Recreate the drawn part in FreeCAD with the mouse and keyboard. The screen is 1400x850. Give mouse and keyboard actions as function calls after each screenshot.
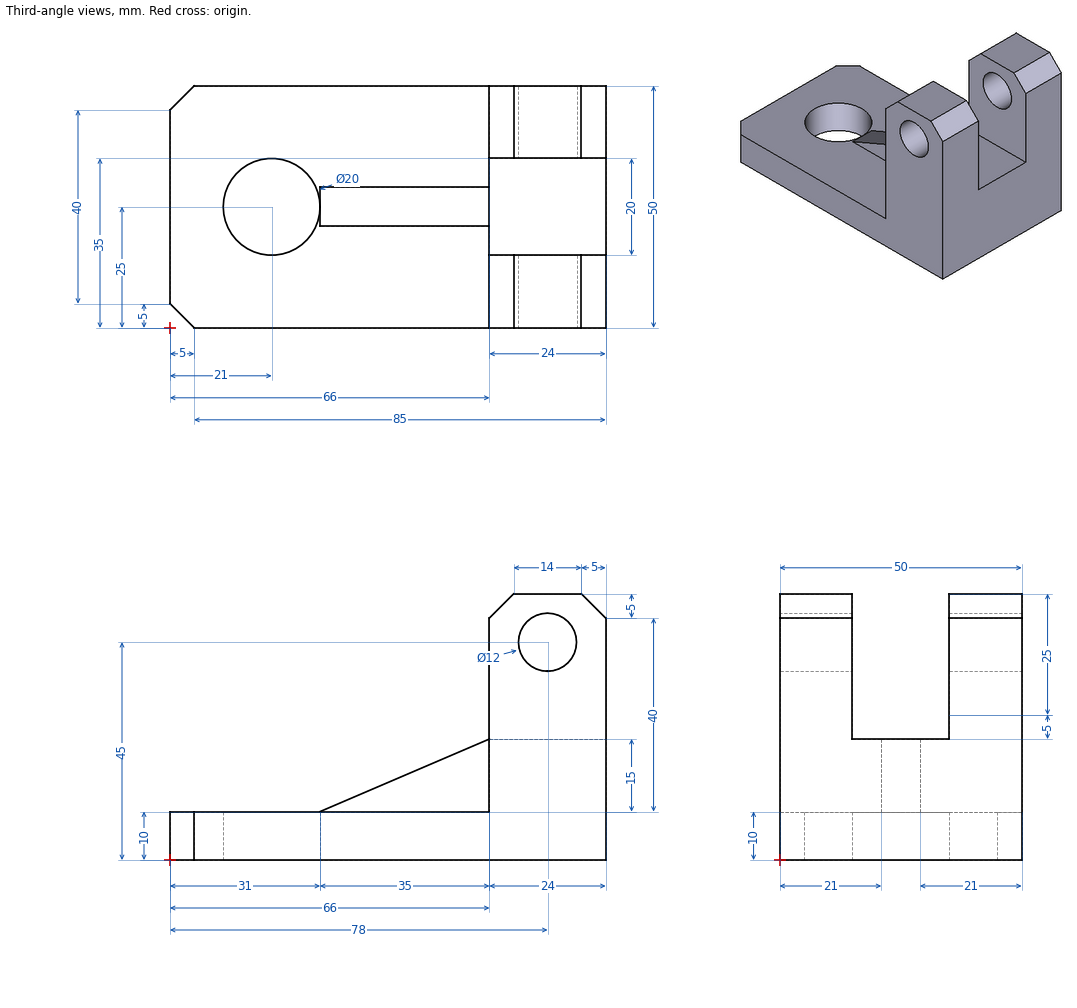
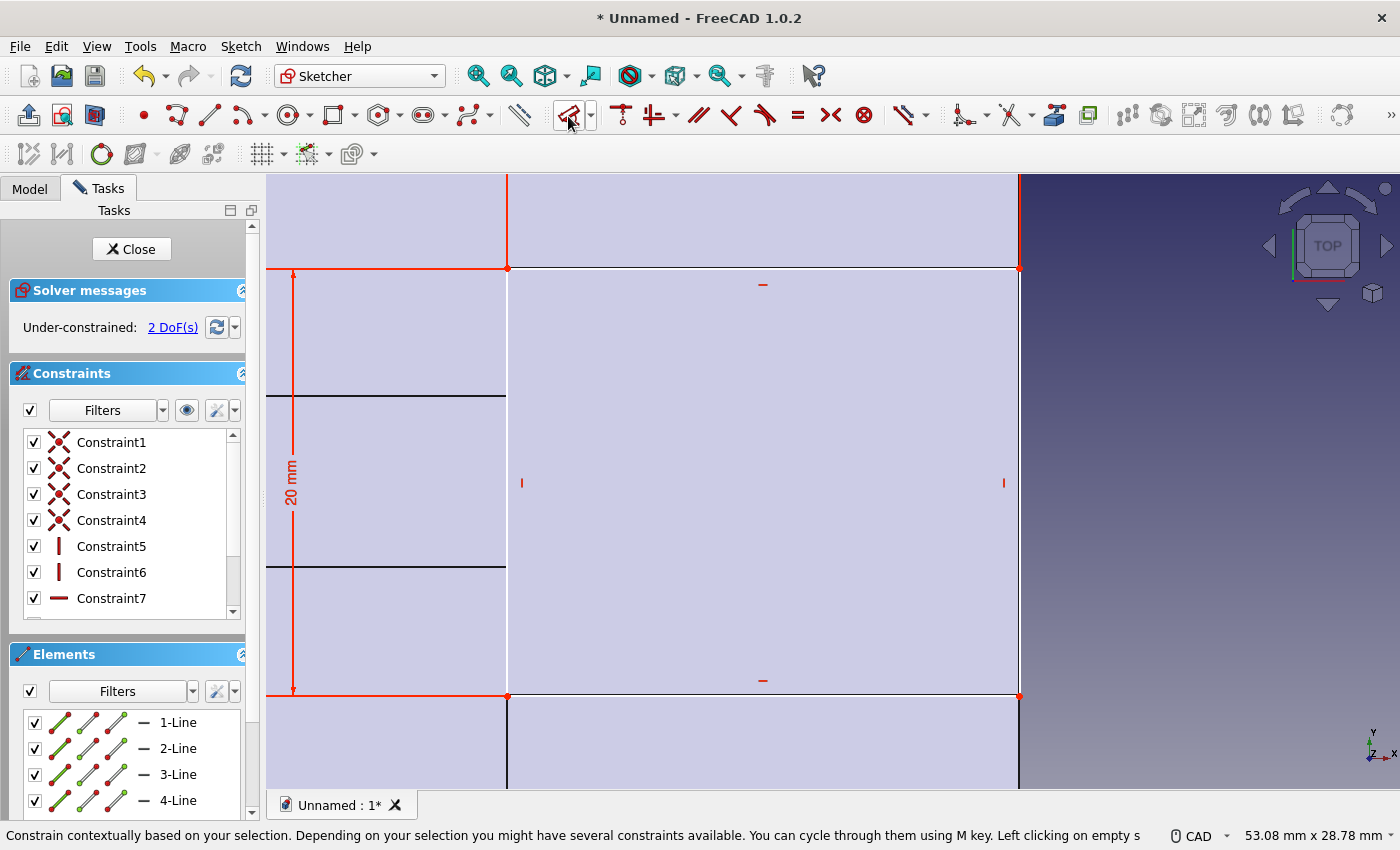
click(507, 269)
click(400, 235)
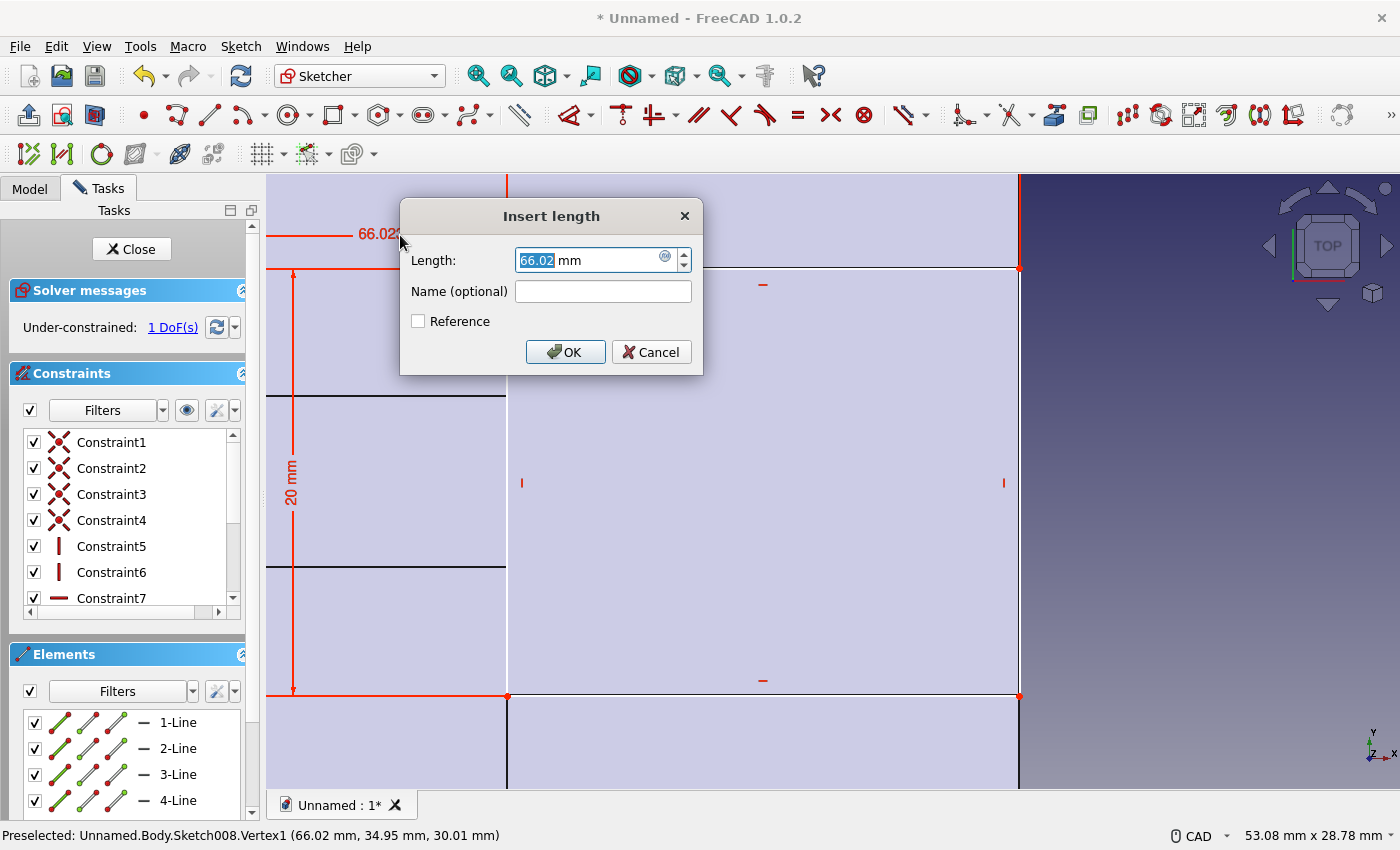
text(66)
key(Return)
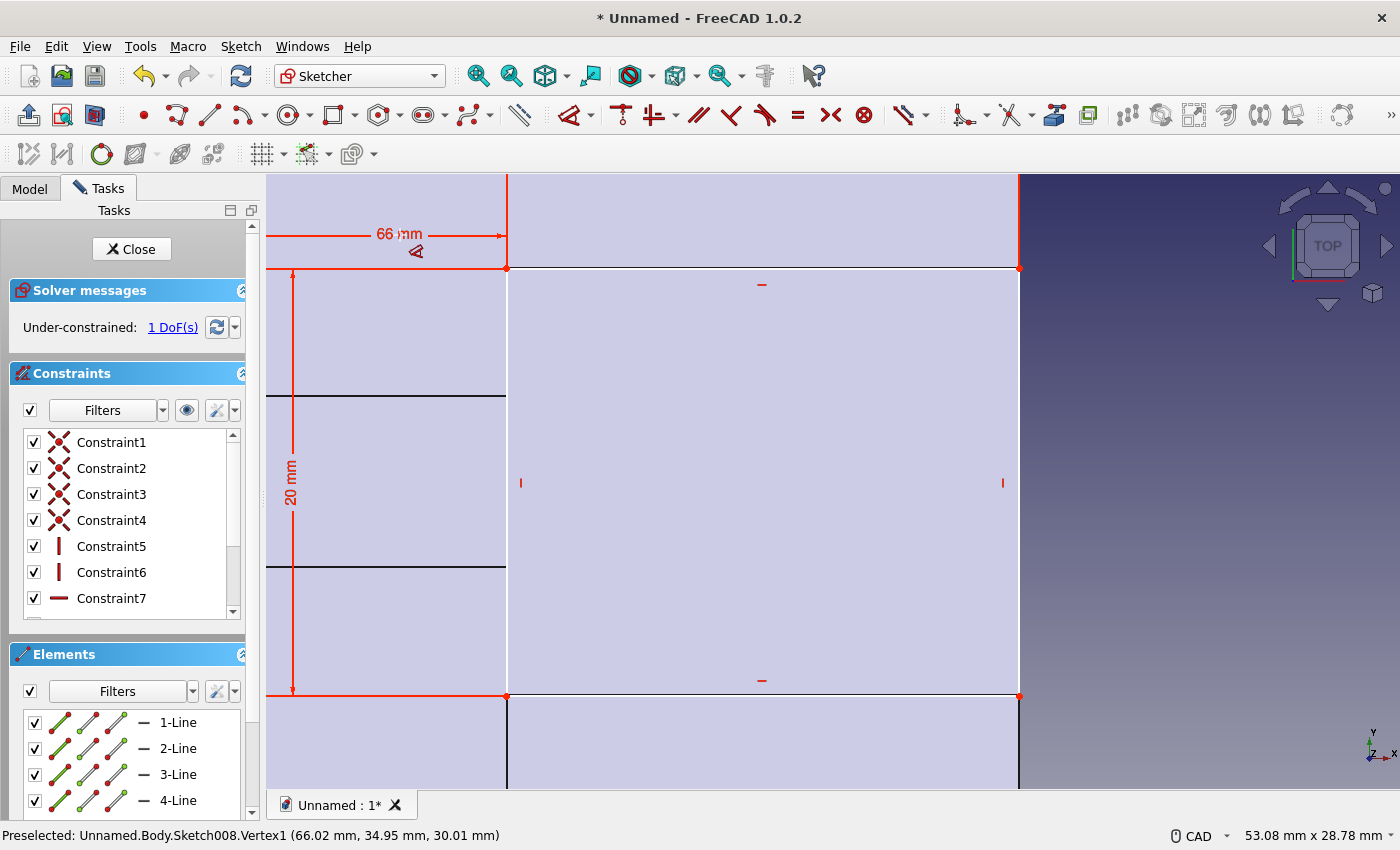
click(507, 269)
click(541, 515)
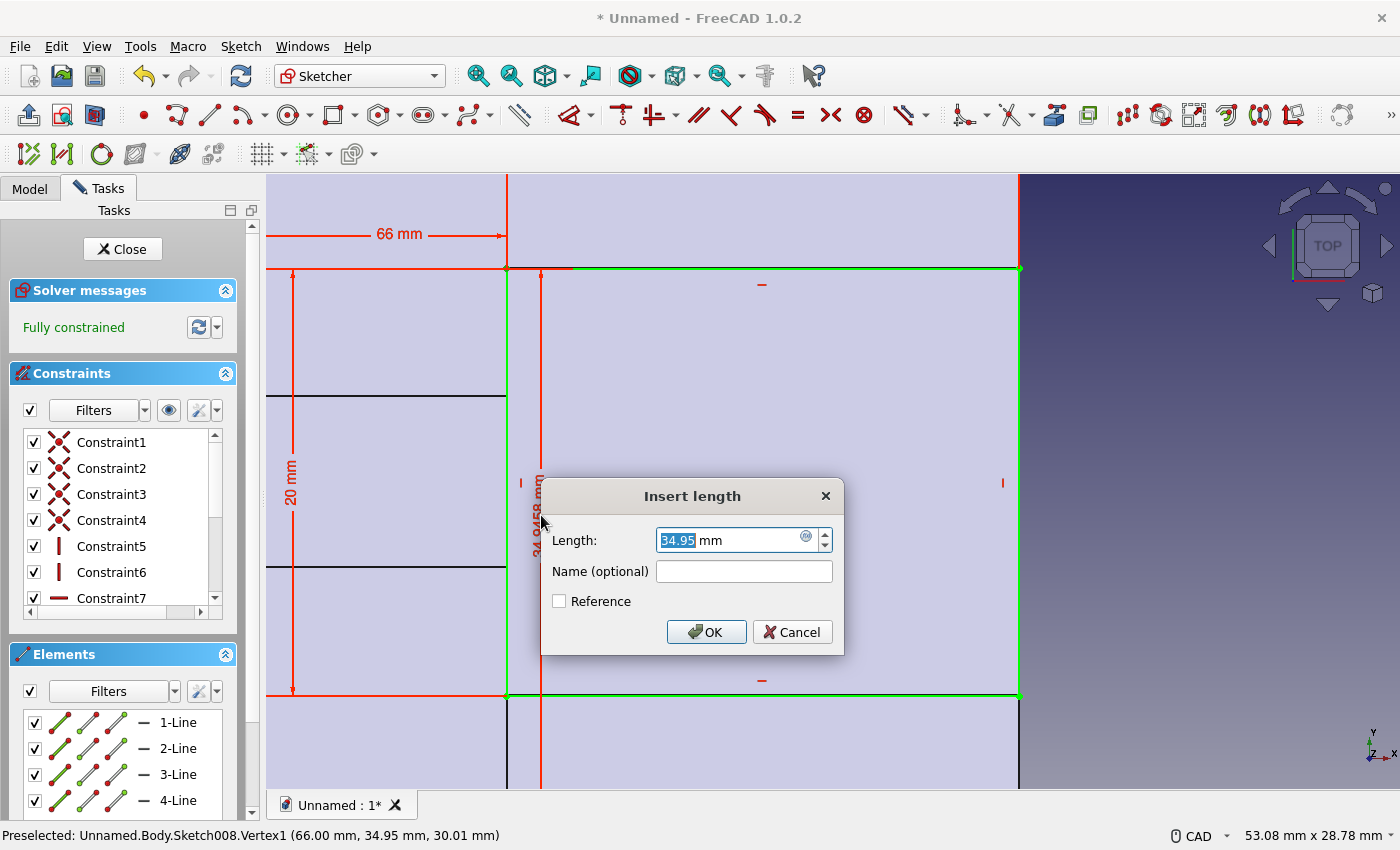
text(35)
key(Return)
key(Escape)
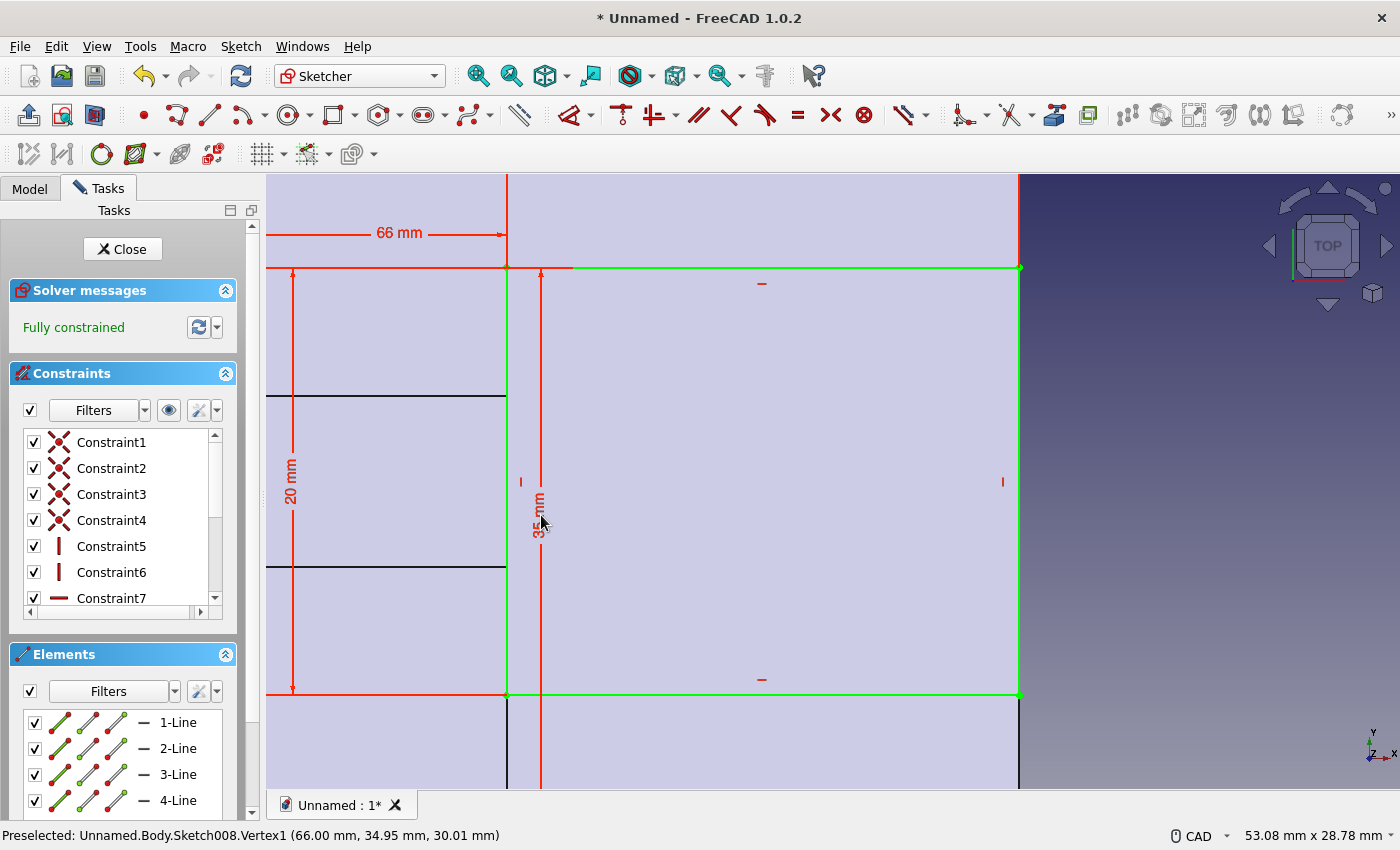
click(123, 249)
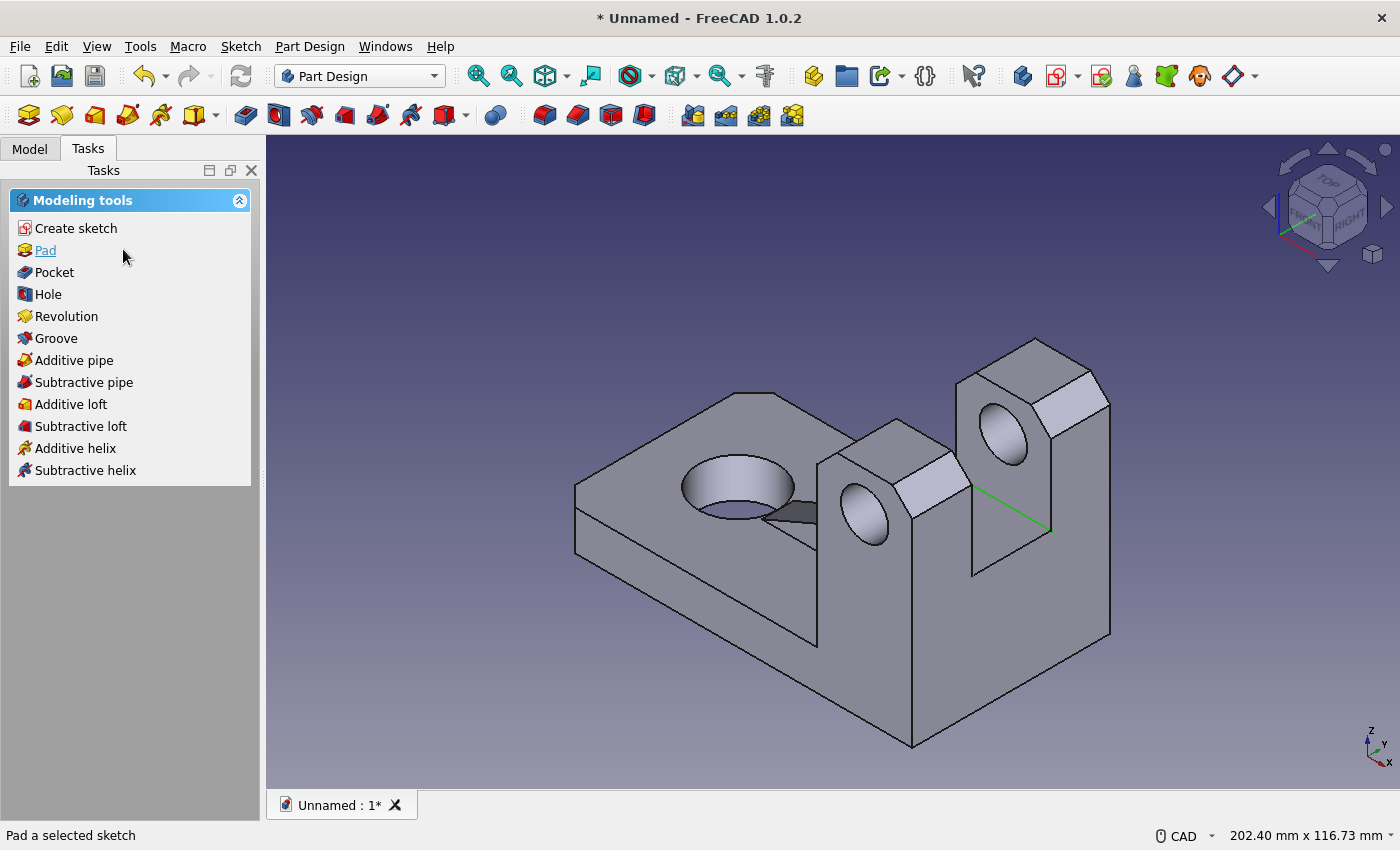
click(246, 116)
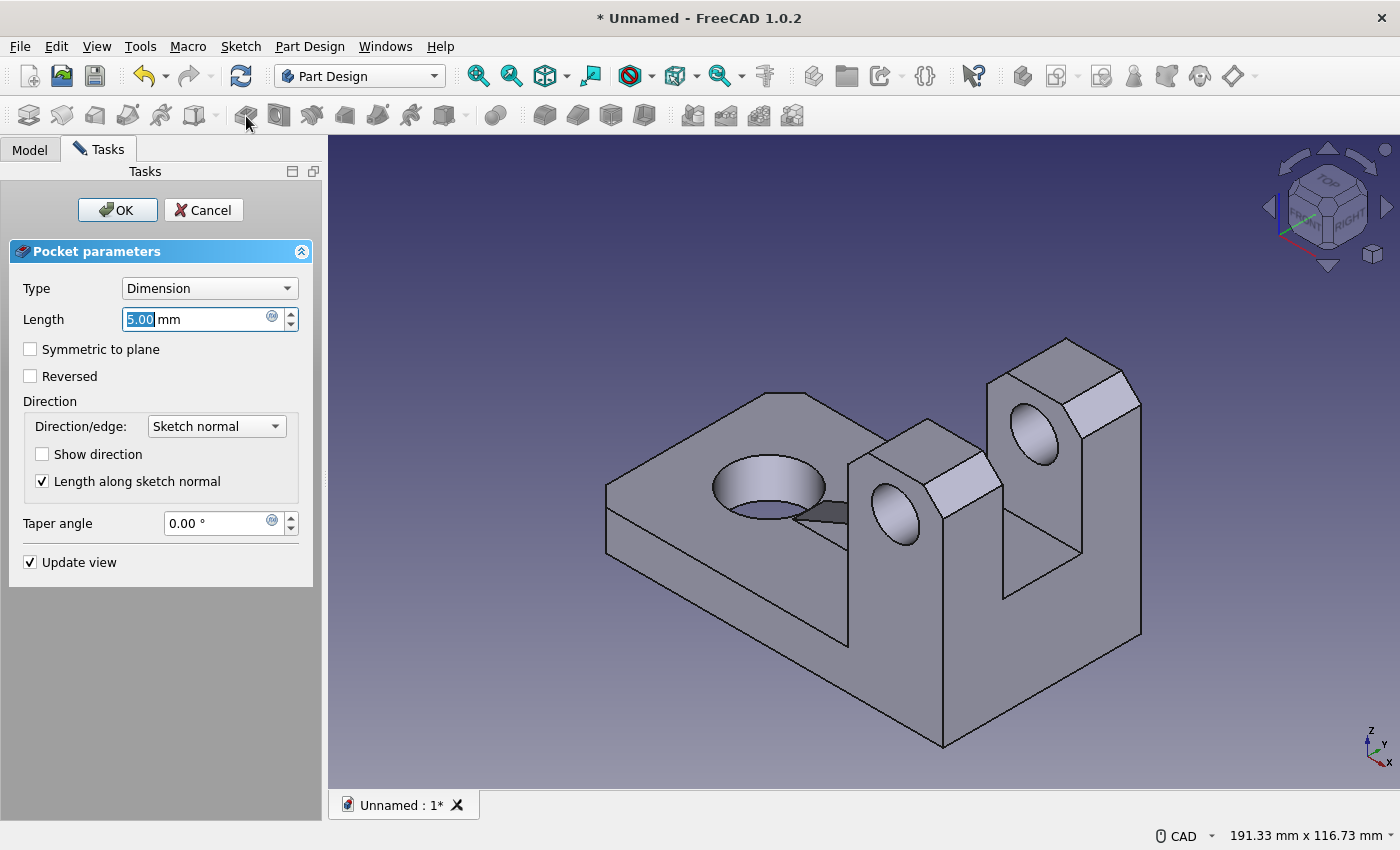
text(5)
key(Tab)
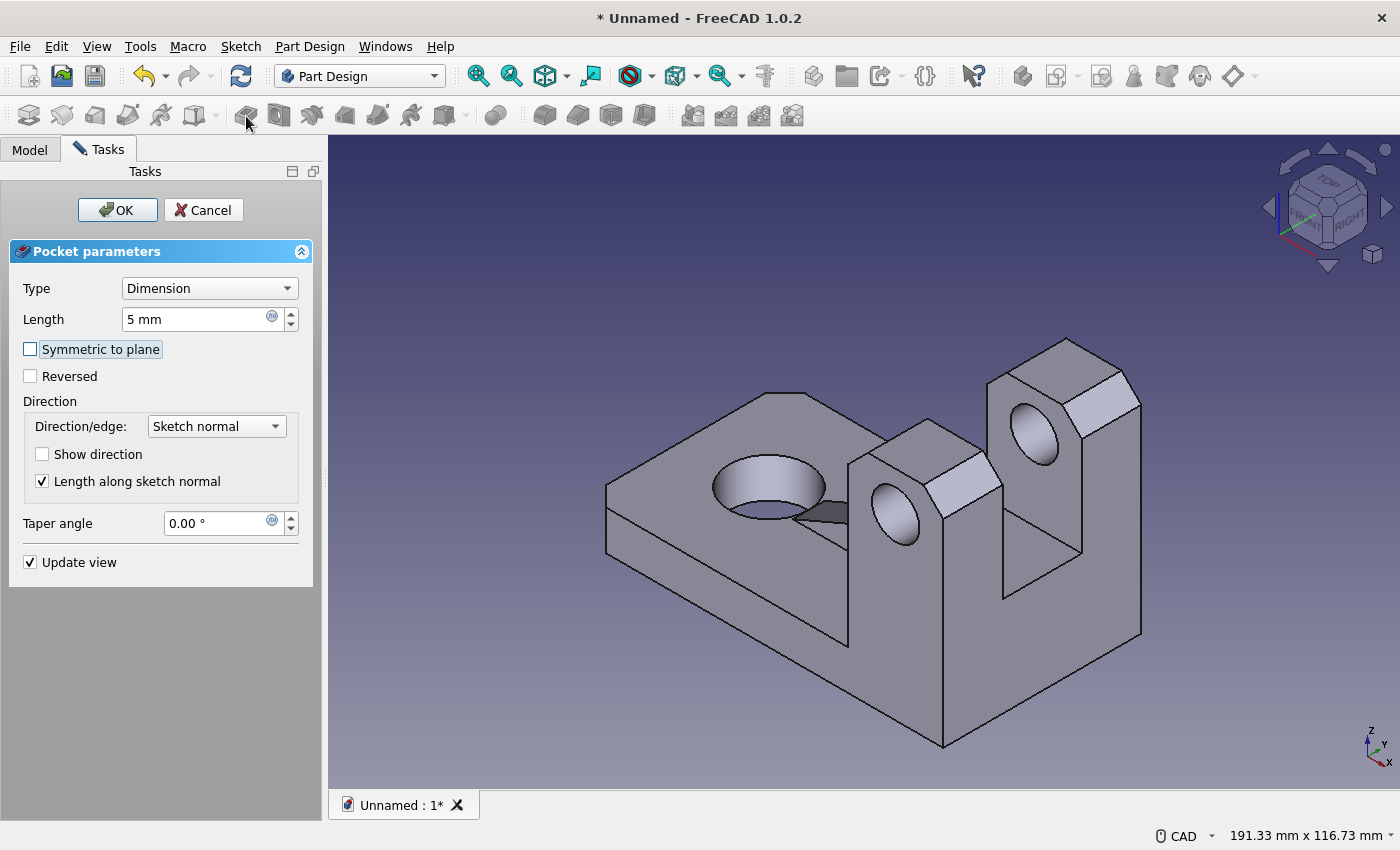
click(118, 210)